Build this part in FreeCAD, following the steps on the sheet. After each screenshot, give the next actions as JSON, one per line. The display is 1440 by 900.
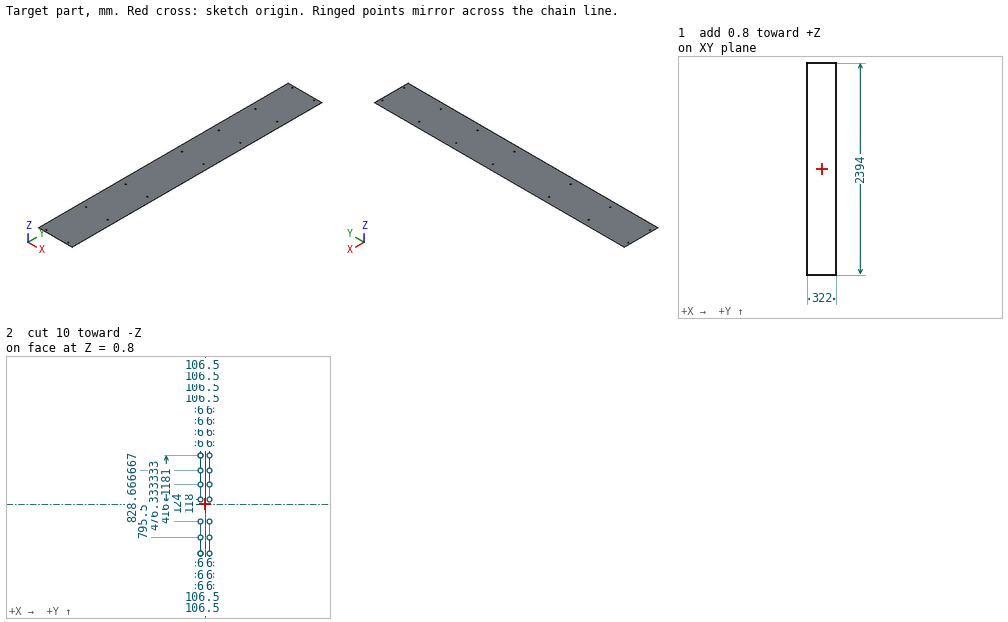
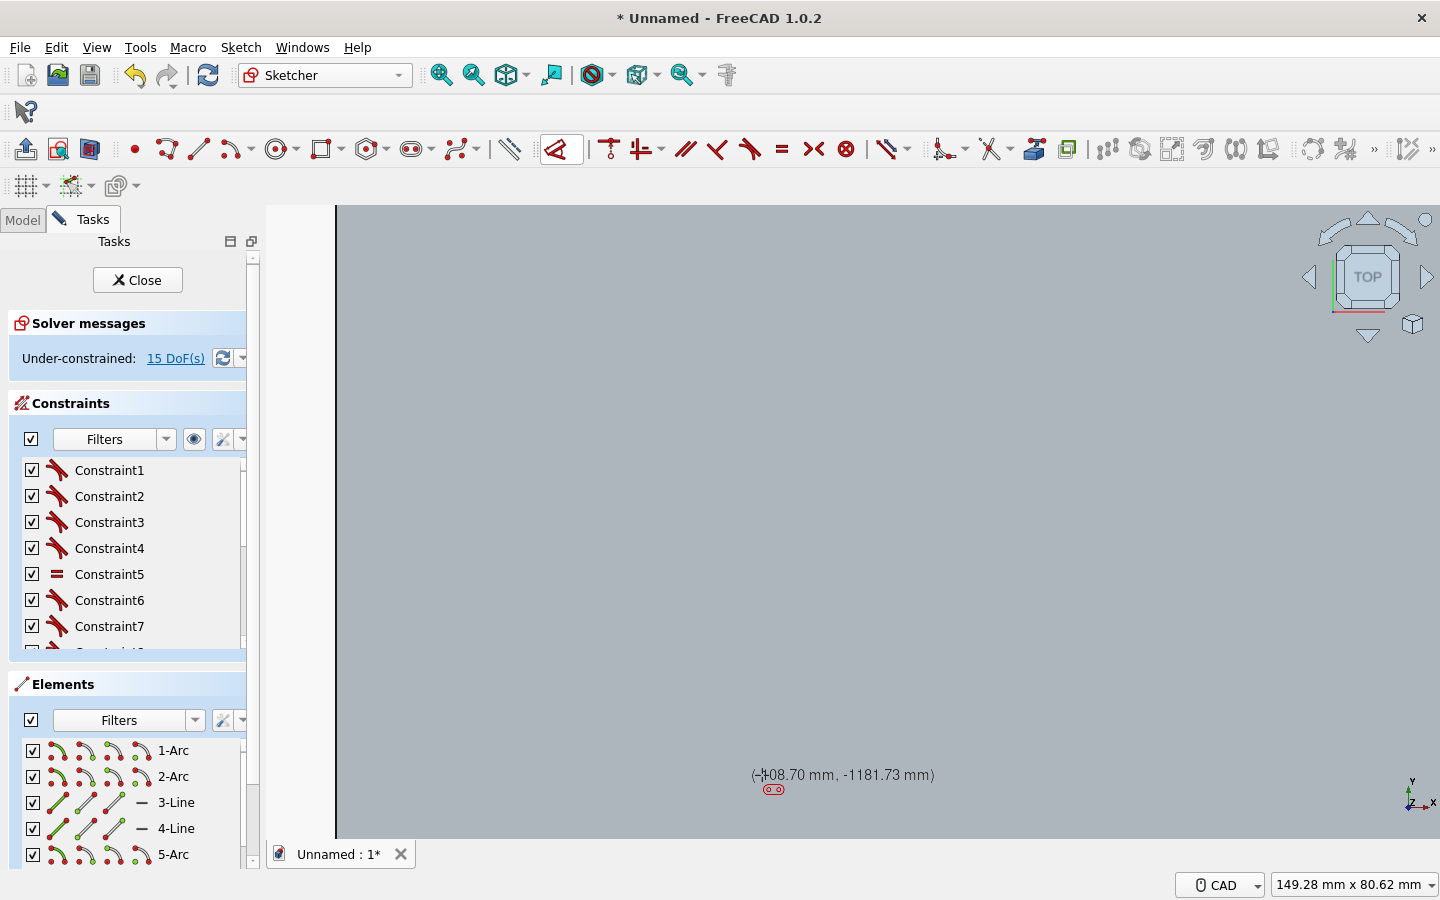
{"action": "scroll", "coordinate": [762, 776], "scroll_direction": "down", "scroll_amount": 18}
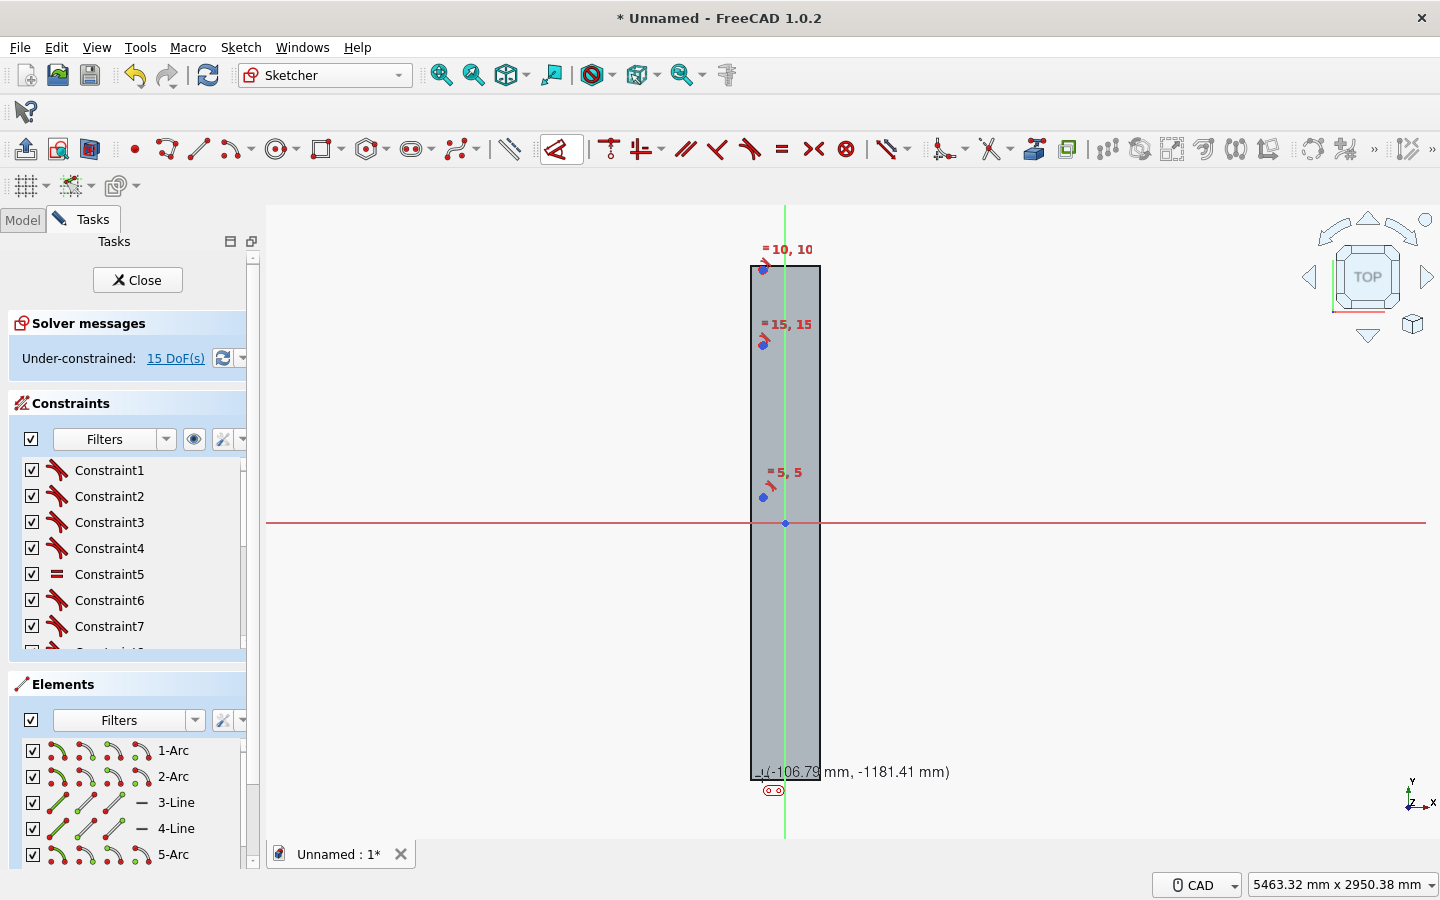
{"action": "left_click", "coordinate": [762, 776]}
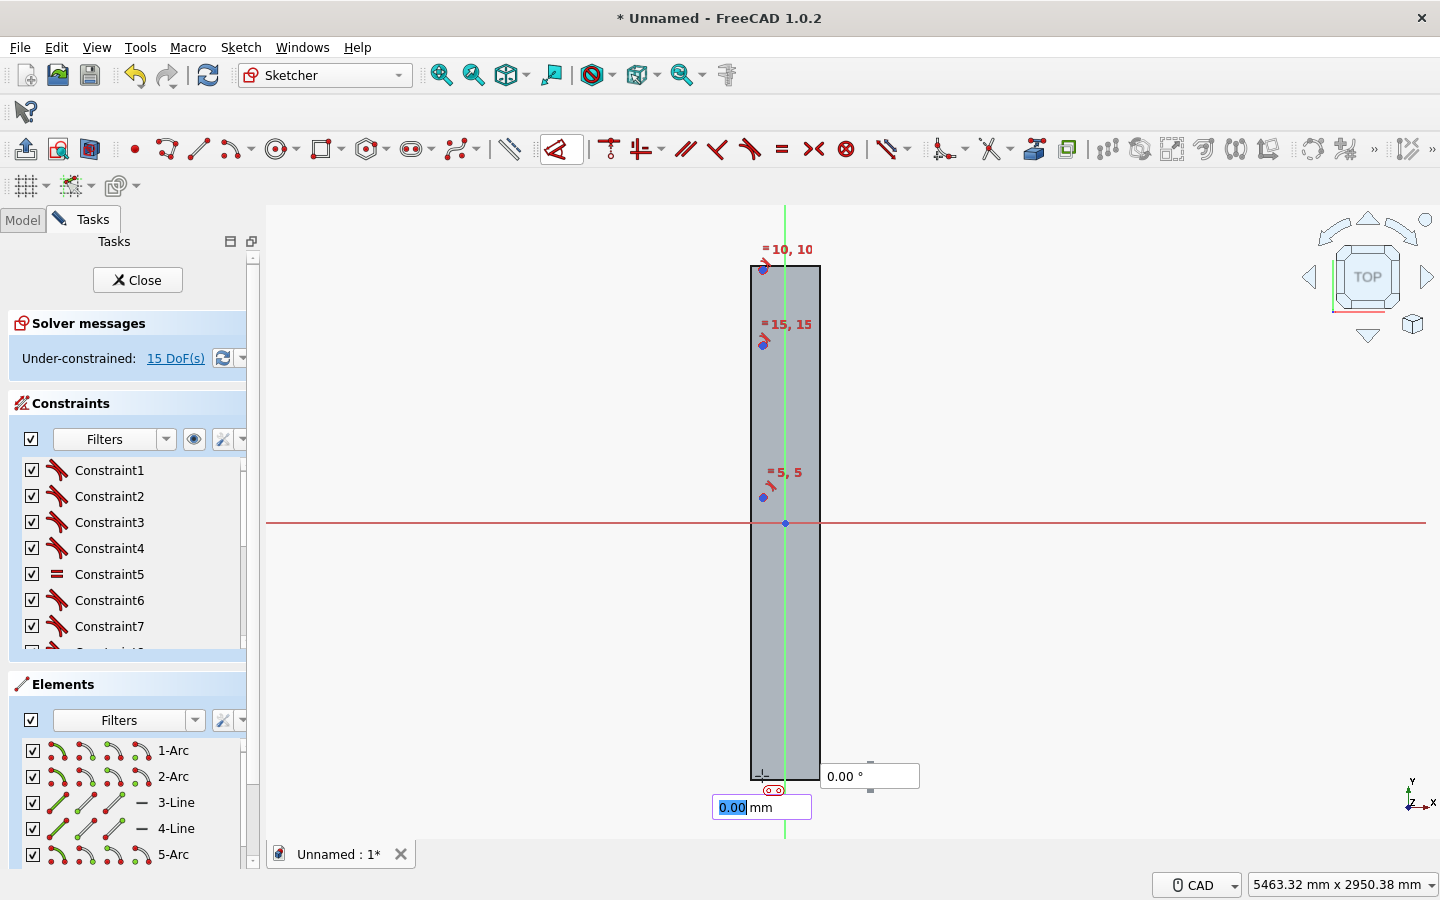
{"action": "scroll", "coordinate": [764, 776], "scroll_direction": "up", "scroll_amount": 13}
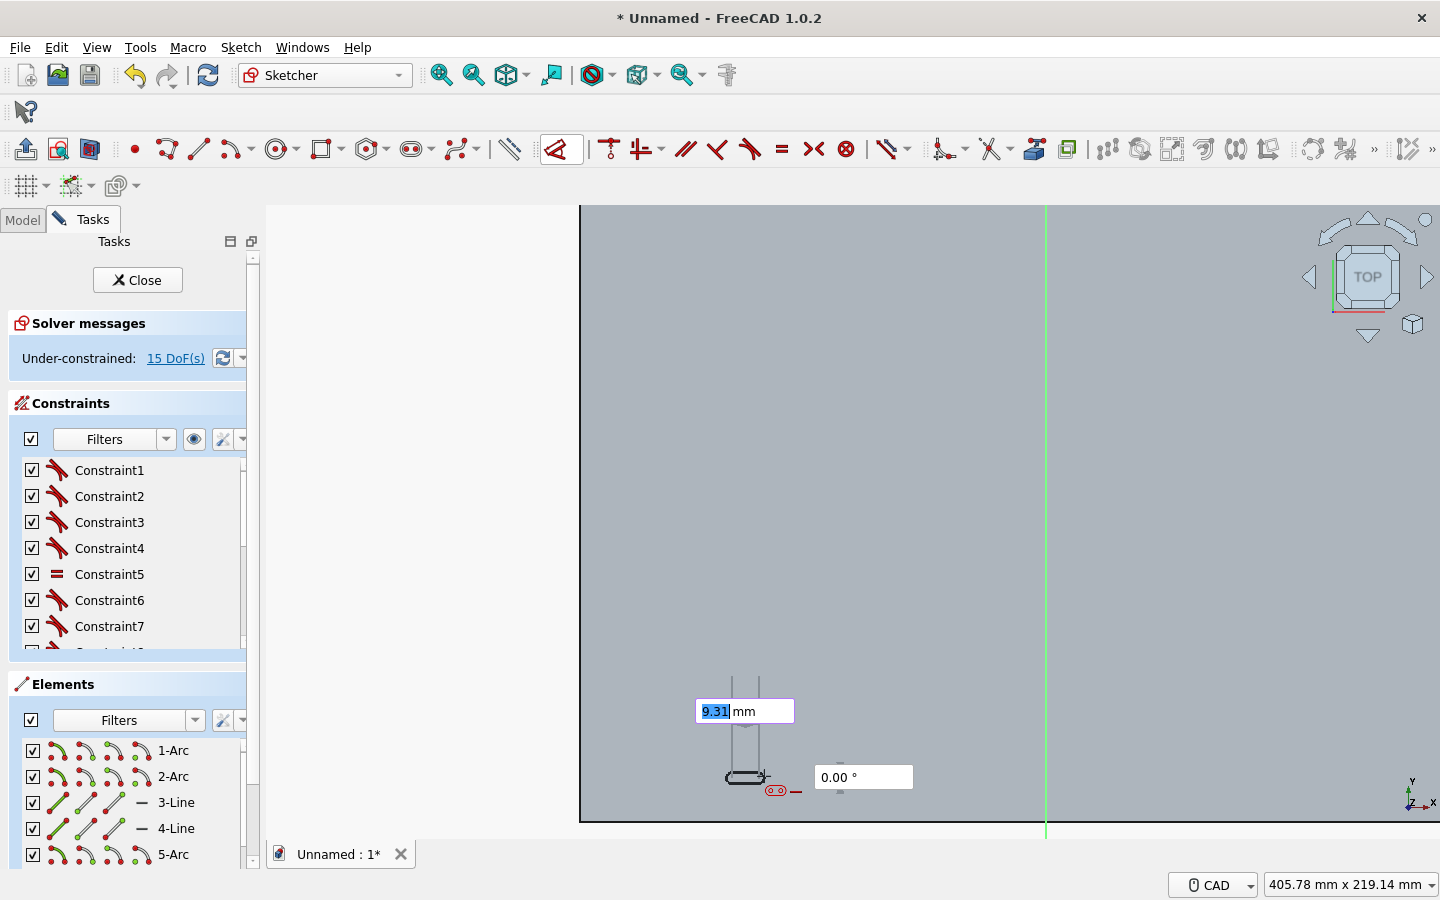
{"action": "left_click", "coordinate": [756, 765]}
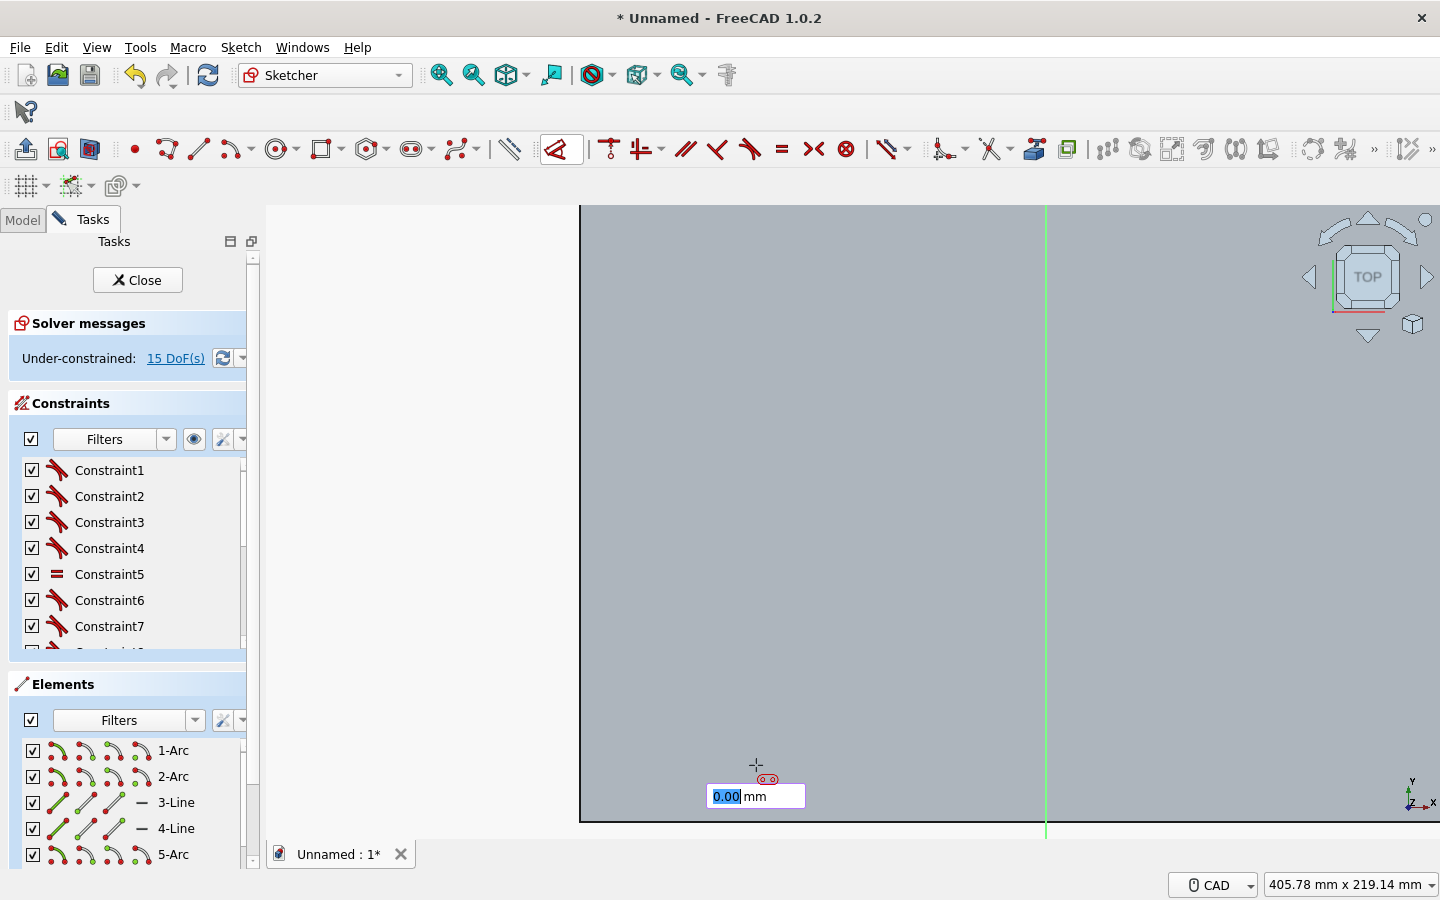
{"action": "scroll", "coordinate": [747, 758], "scroll_direction": "up", "scroll_amount": 4}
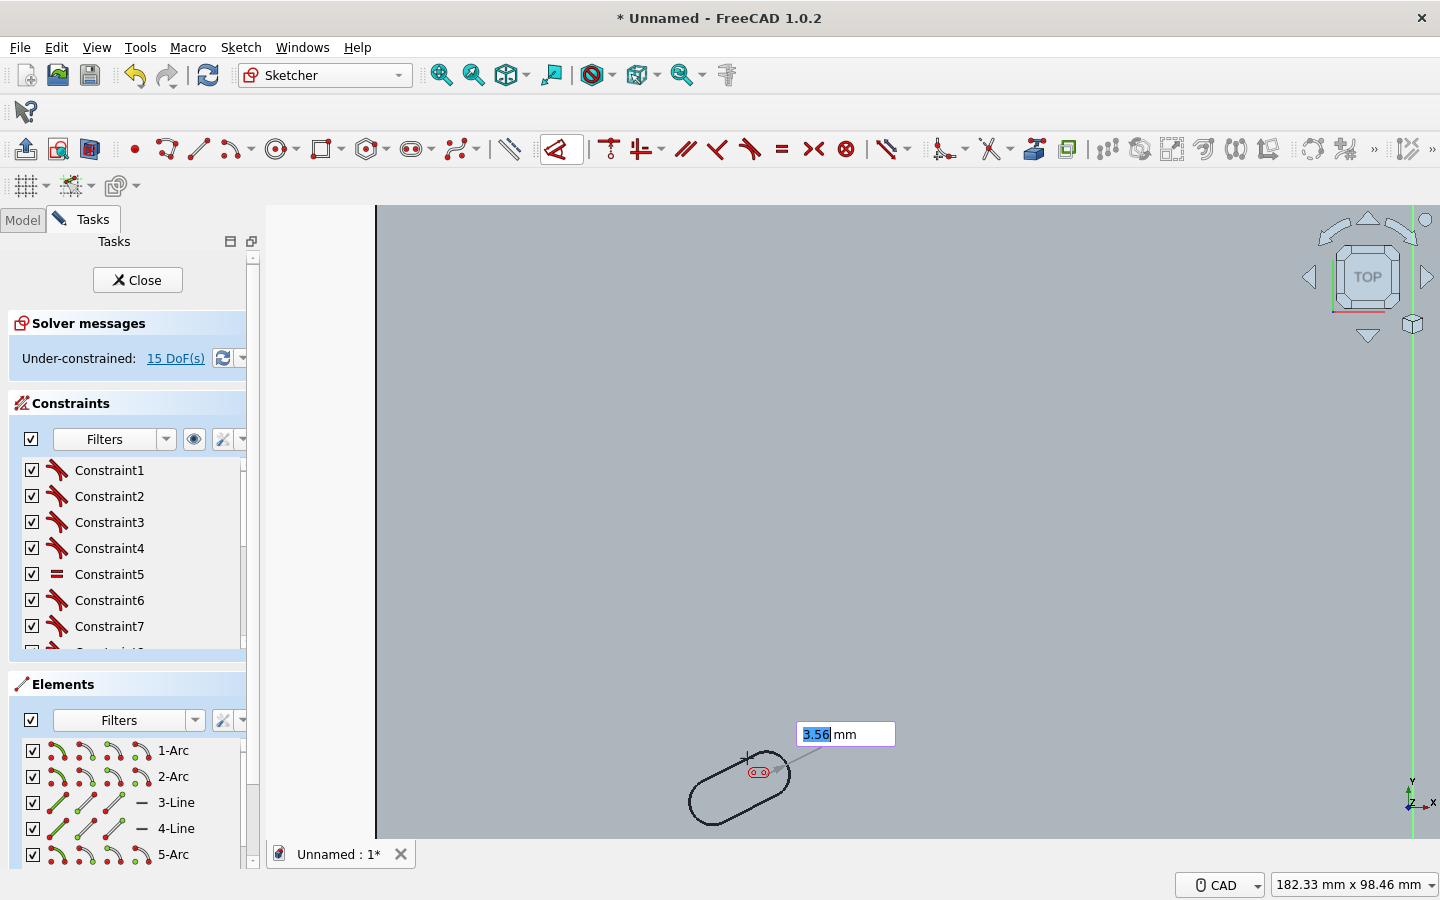
{"action": "left_click", "coordinate": [746, 758]}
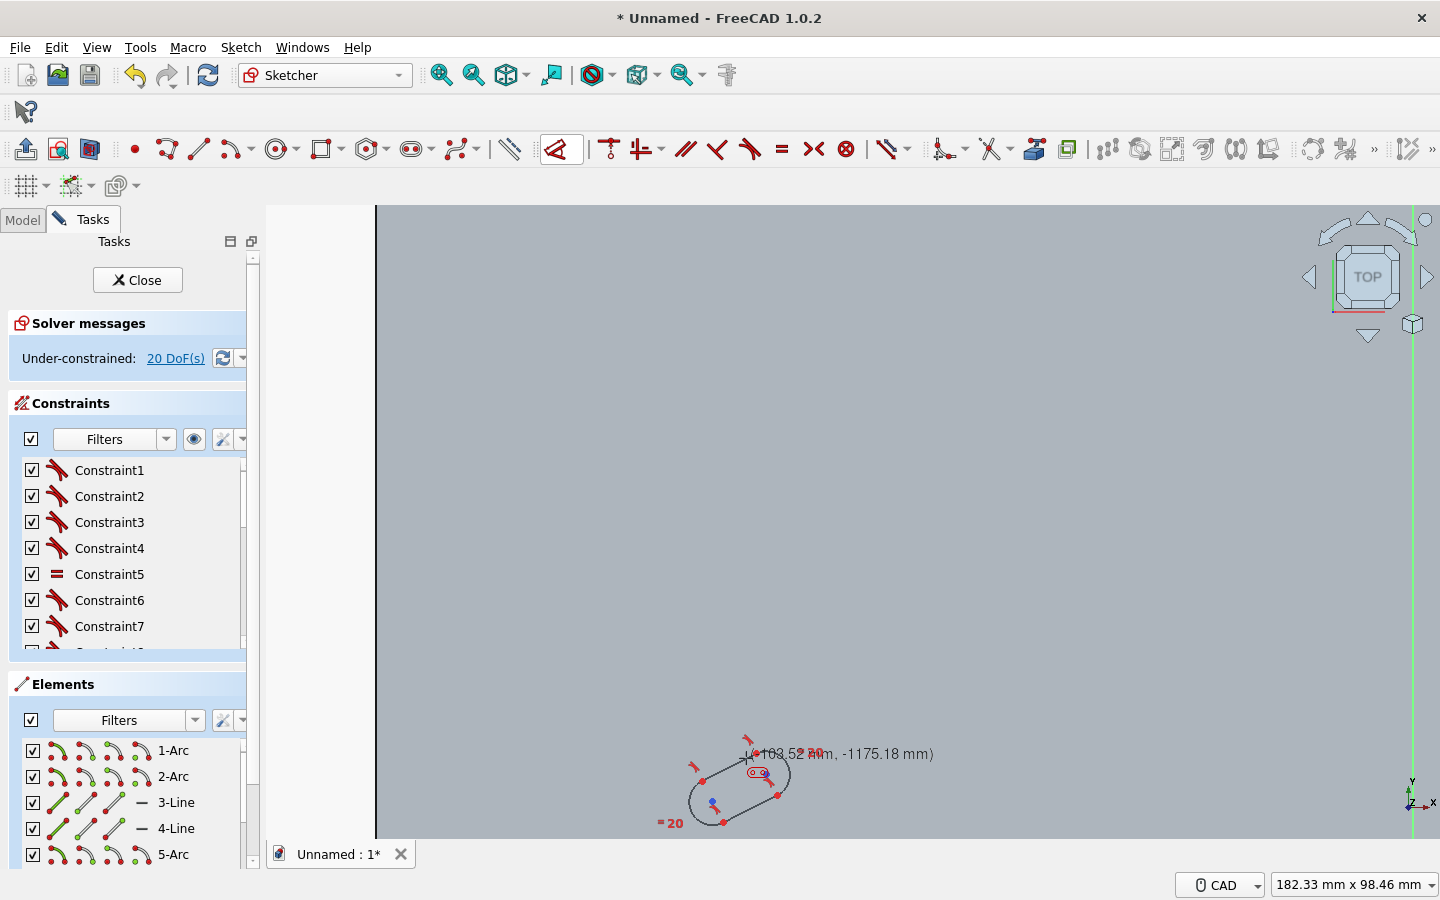
{"action": "scroll", "coordinate": [763, 775], "scroll_direction": "down", "scroll_amount": 17}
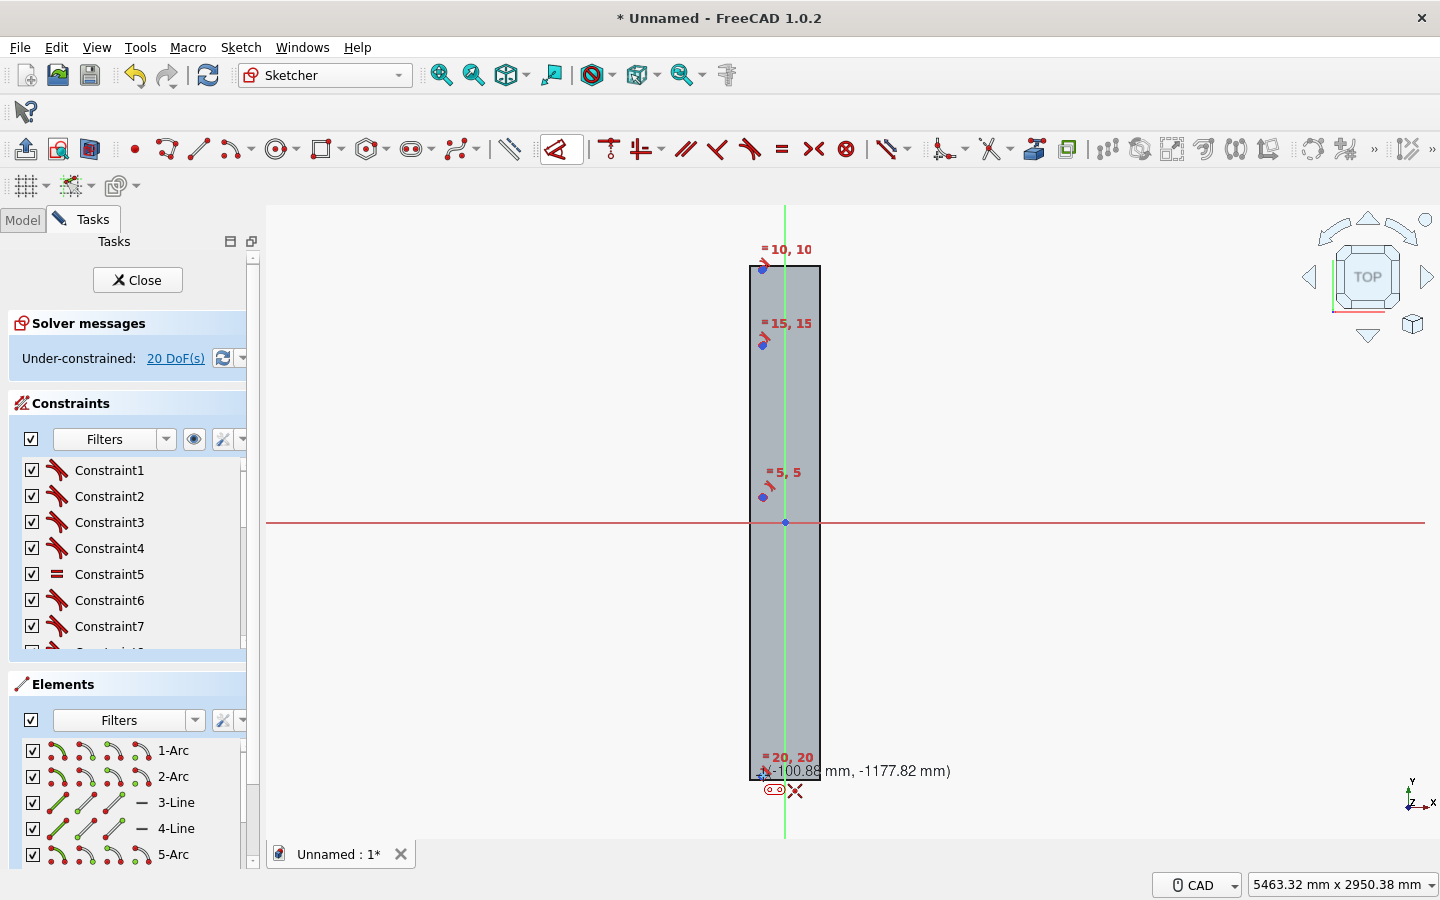
{"action": "scroll", "coordinate": [762, 421], "scroll_direction": "up", "scroll_amount": 18}